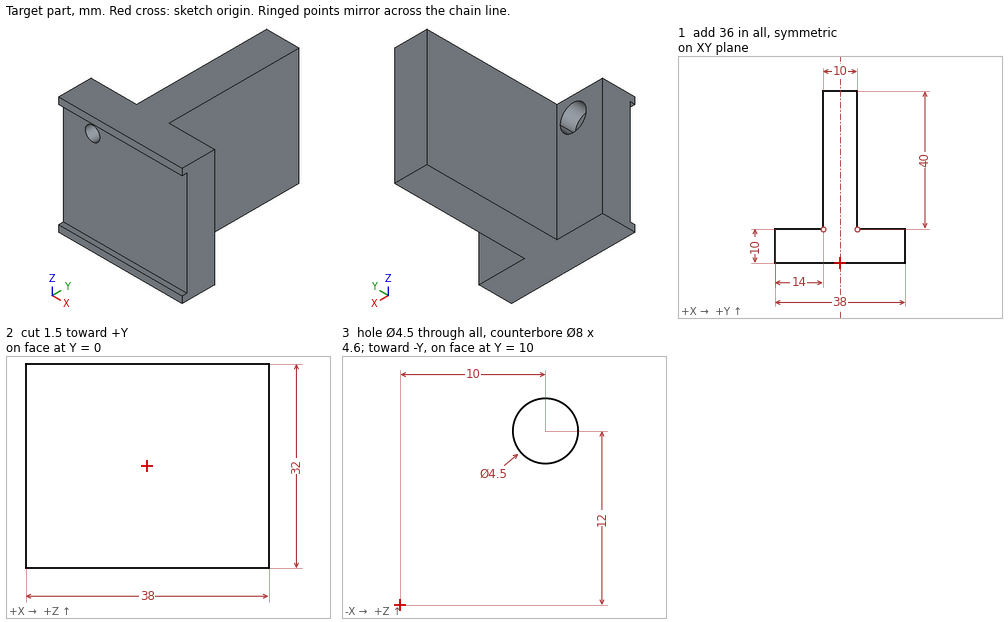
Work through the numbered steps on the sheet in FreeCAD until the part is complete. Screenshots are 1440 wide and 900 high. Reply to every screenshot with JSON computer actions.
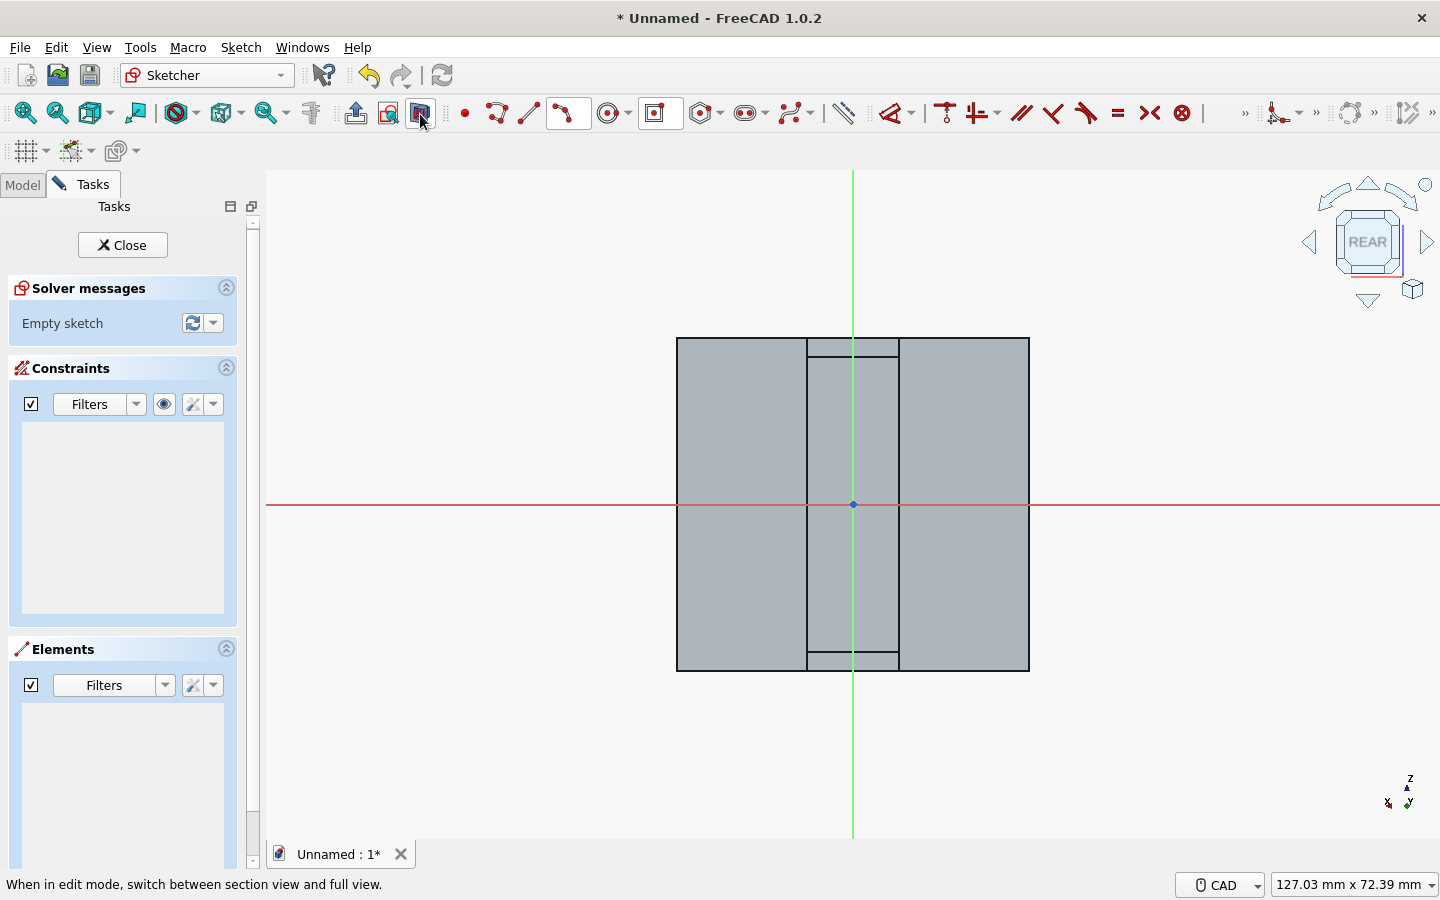
{"action": "scroll", "coordinate": [961, 383], "scroll_direction": "up", "scroll_amount": 12}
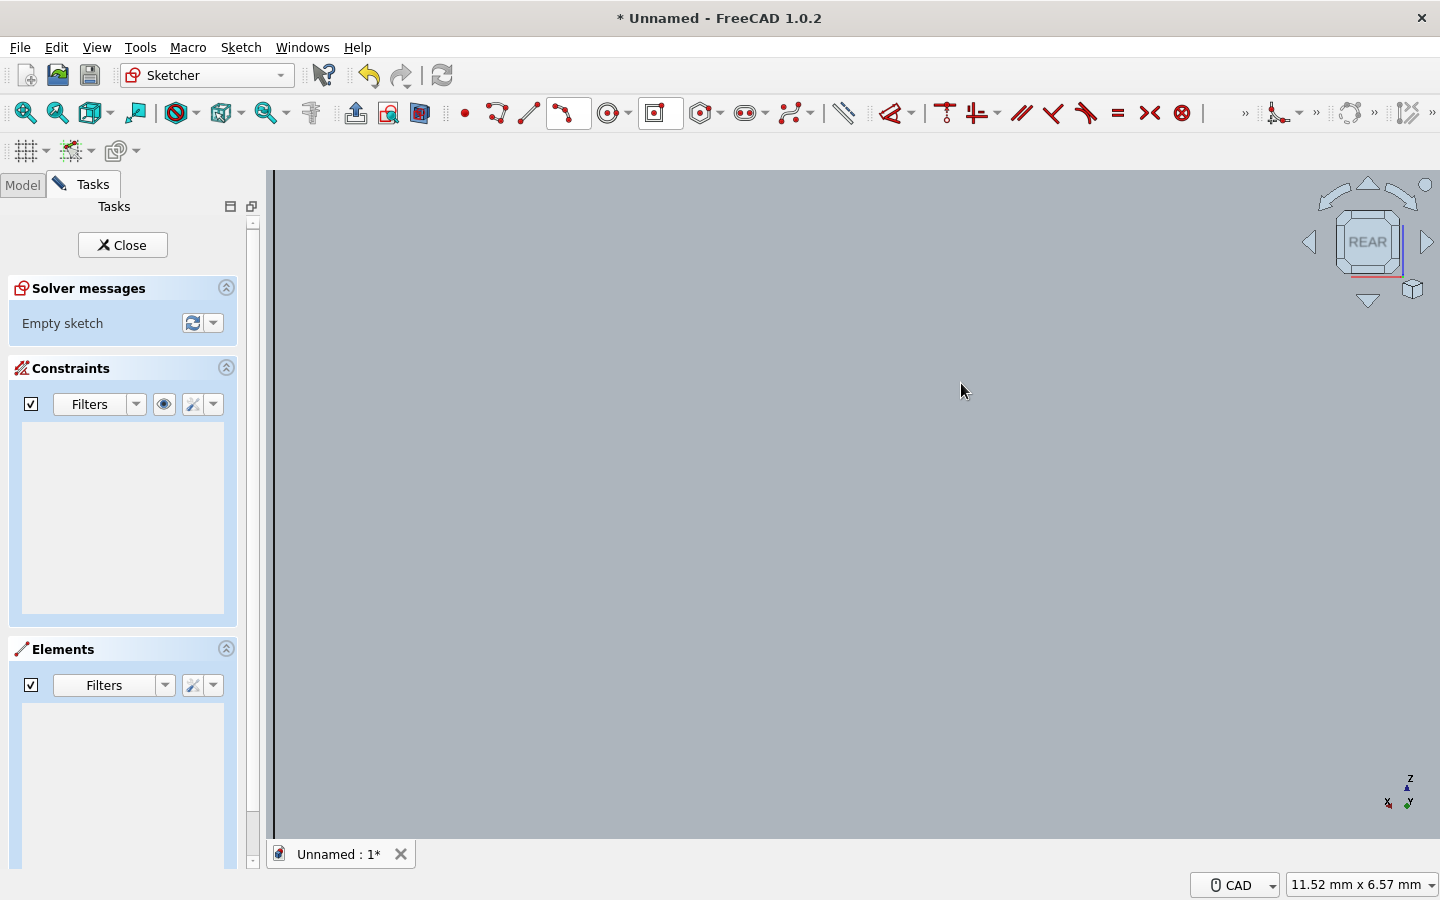
{"action": "left_click", "coordinate": [608, 114]}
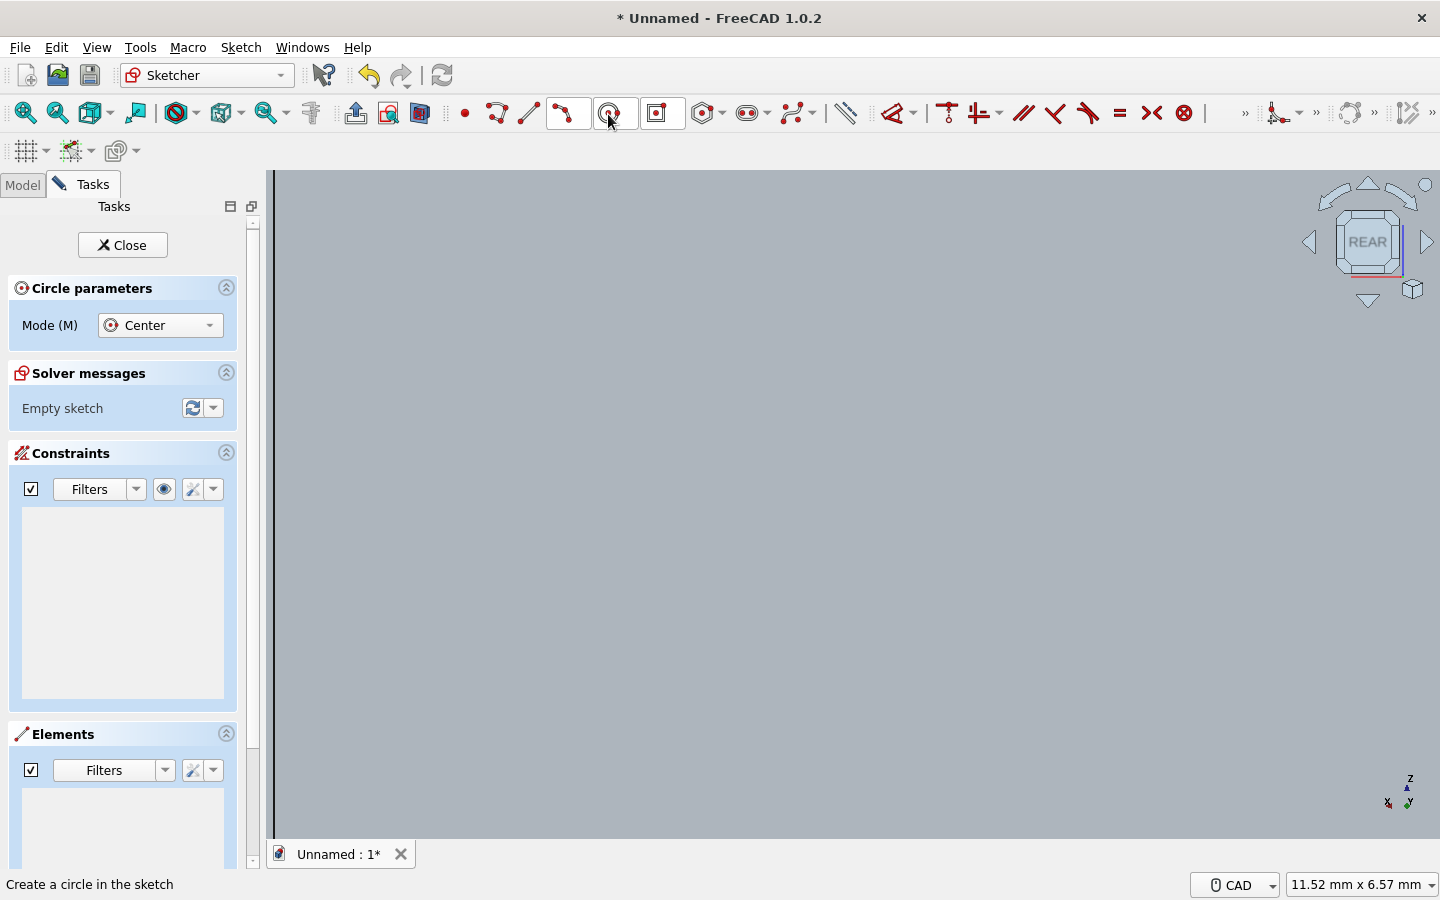
{"action": "left_click", "coordinate": [783, 497]}
{"action": "left_click", "coordinate": [945, 335]}
{"action": "key", "text": "Escape"}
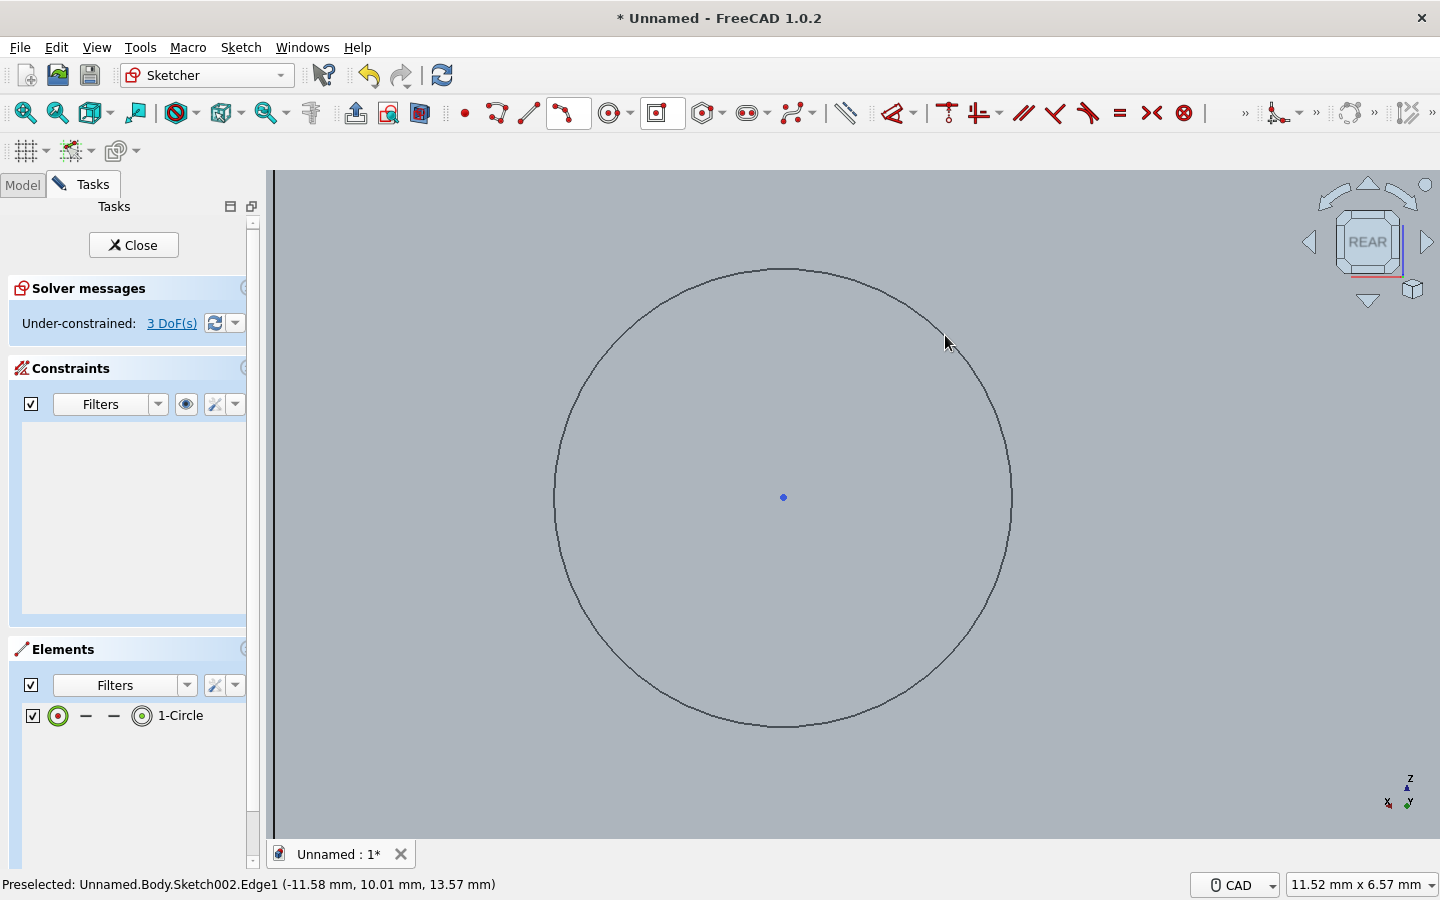
{"action": "left_click", "coordinate": [892, 114]}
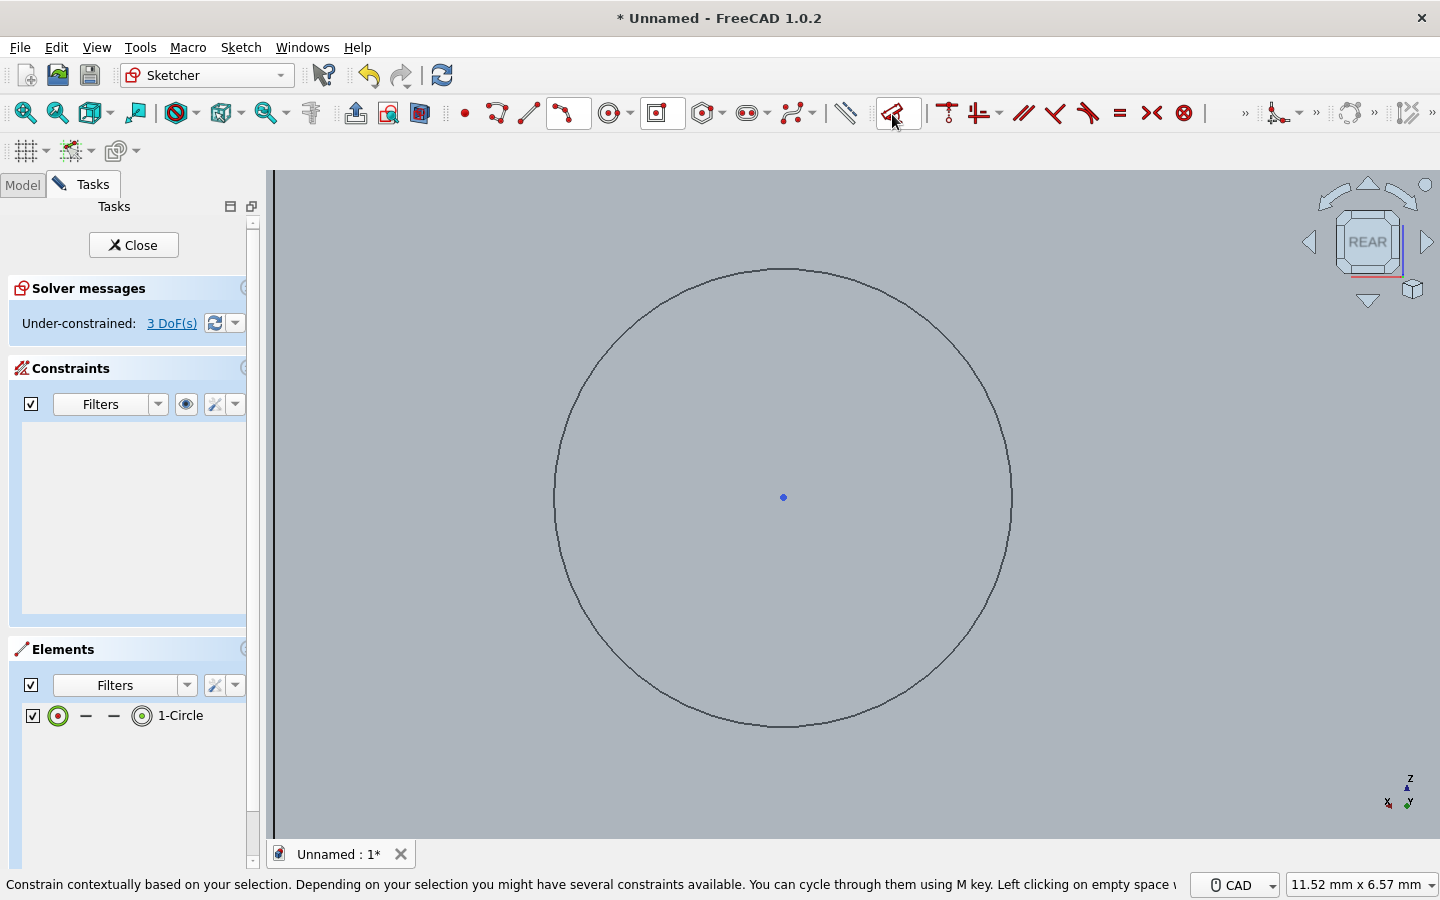
{"action": "left_click", "coordinate": [944, 335]}
{"action": "left_click", "coordinate": [966, 312]}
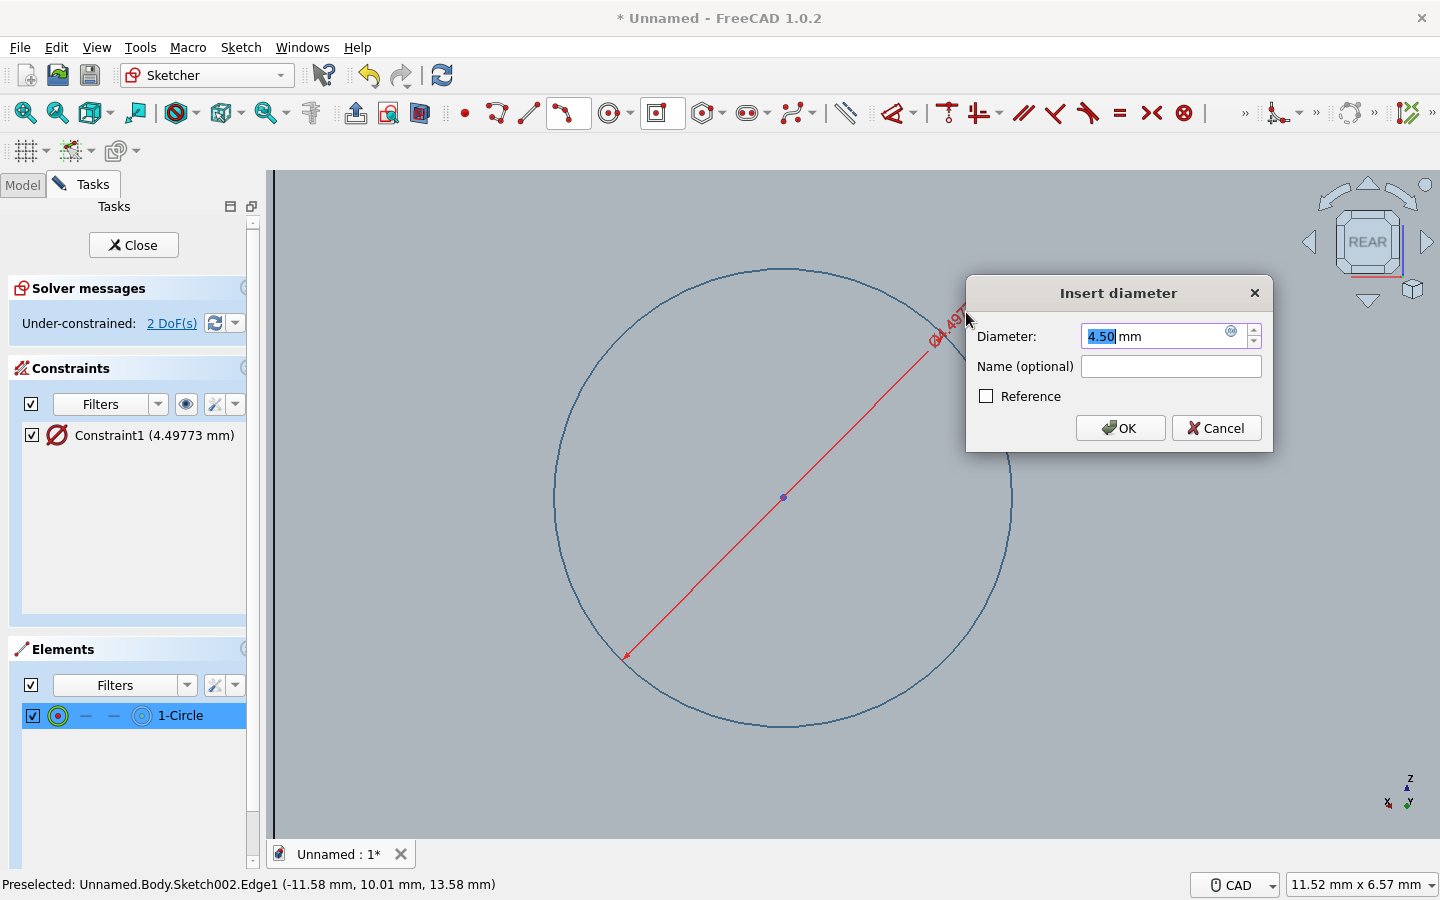
{"action": "type", "text": "4.5"}
{"action": "key", "text": "Return"}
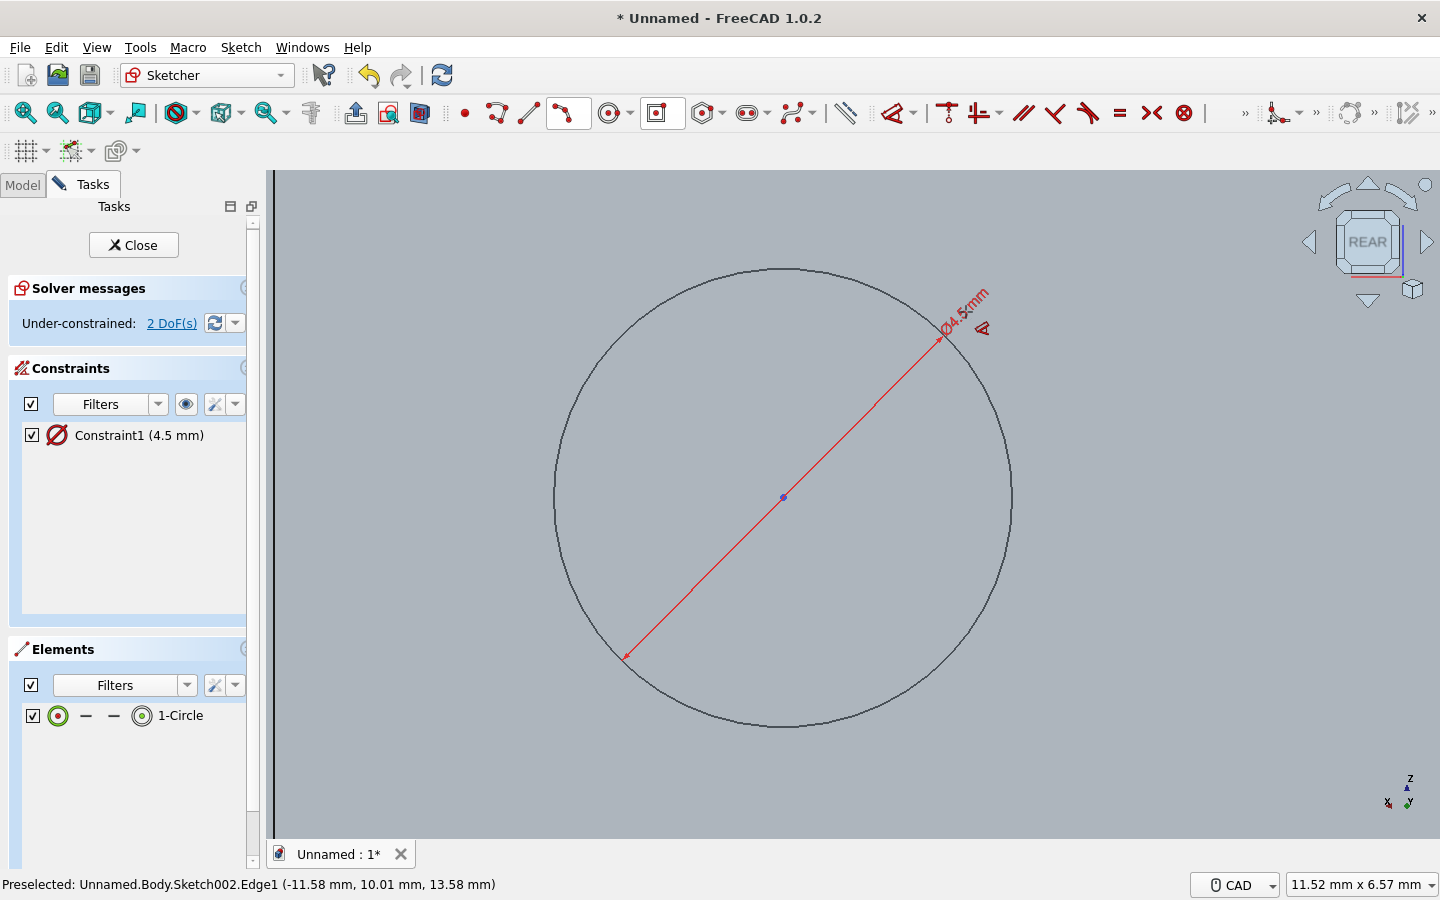
{"action": "left_click", "coordinate": [783, 498]}
{"action": "left_click", "coordinate": [539, 464]}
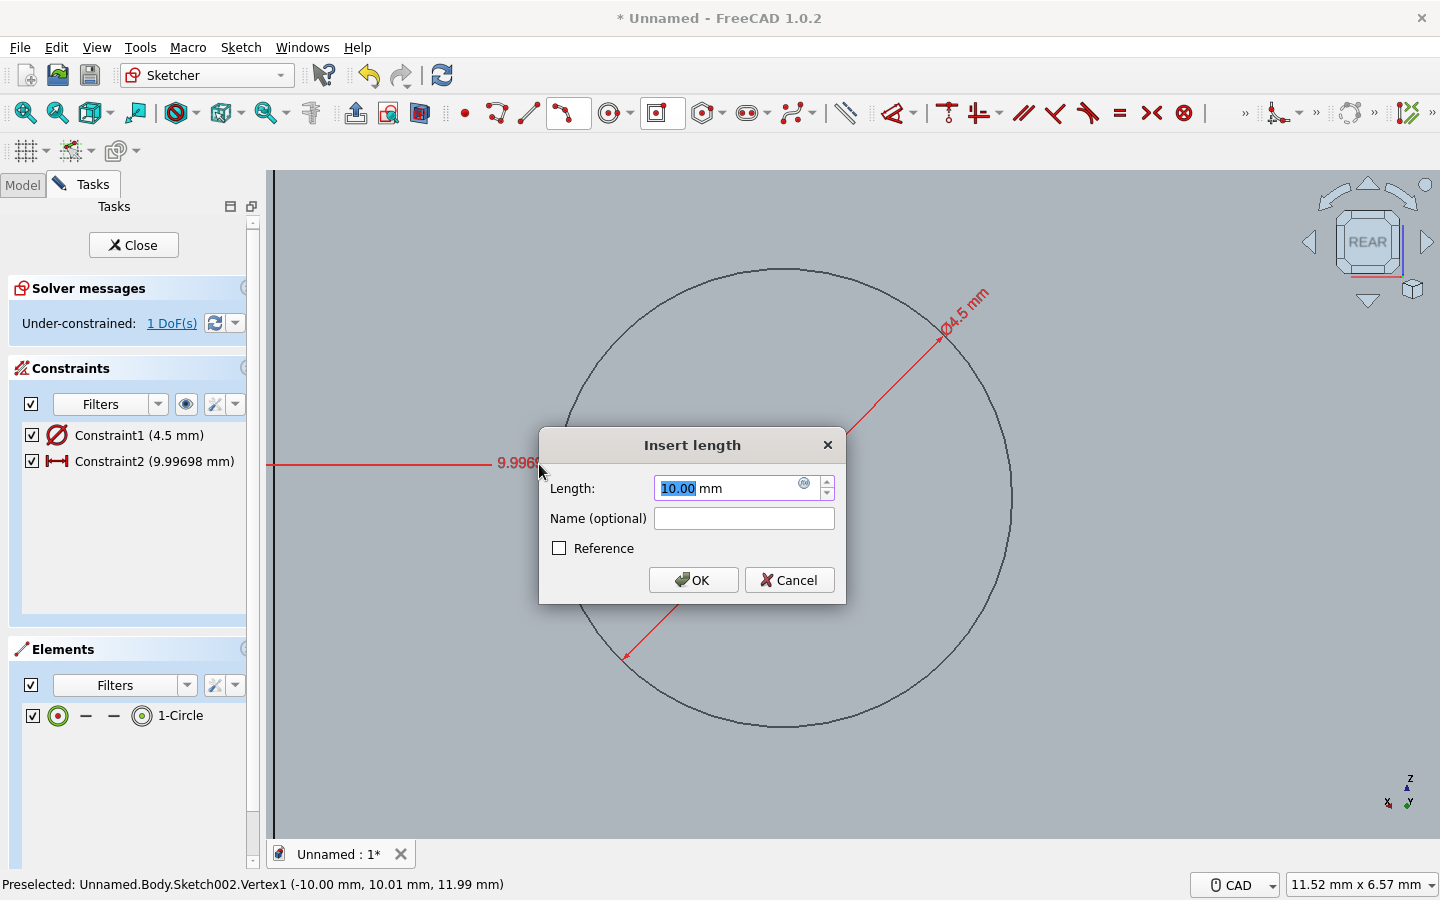
{"action": "type", "text": "10"}
{"action": "key", "text": "Return"}